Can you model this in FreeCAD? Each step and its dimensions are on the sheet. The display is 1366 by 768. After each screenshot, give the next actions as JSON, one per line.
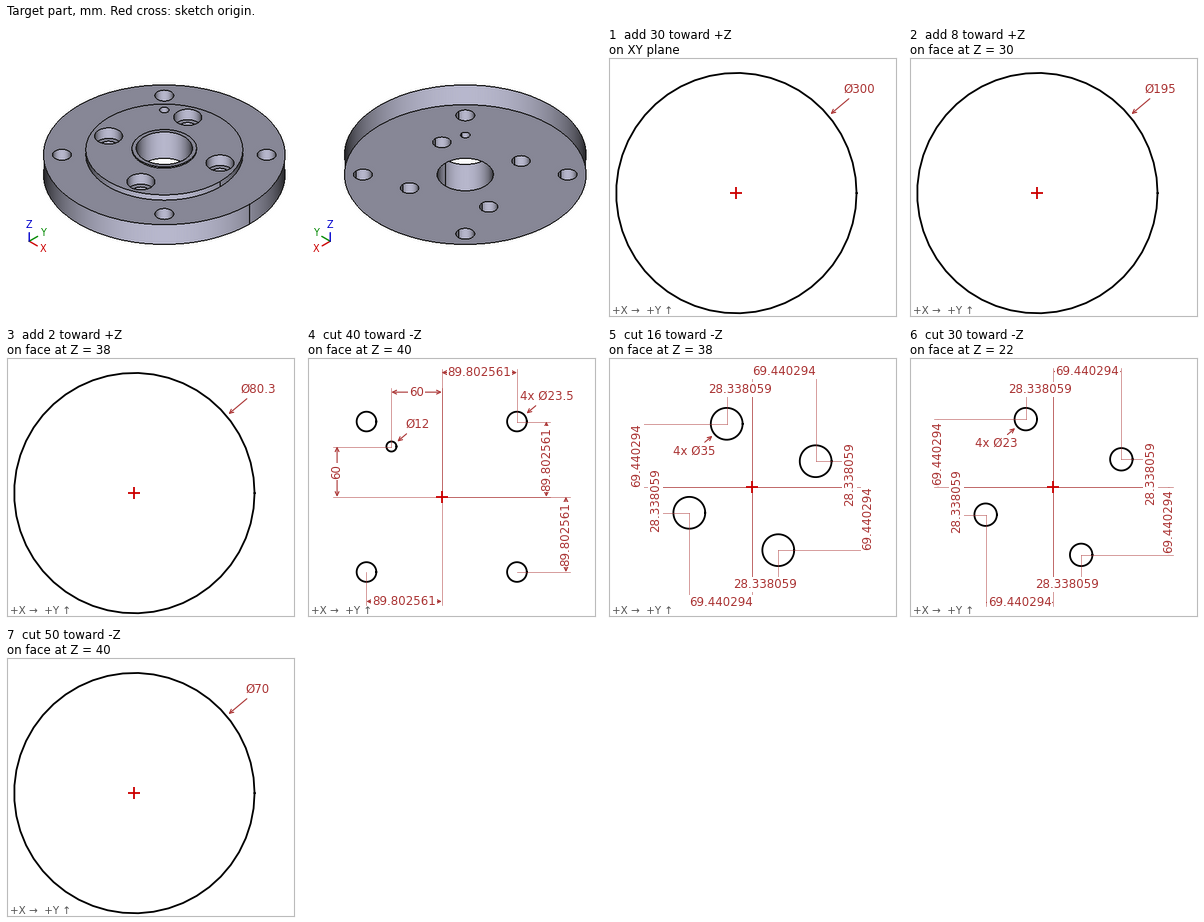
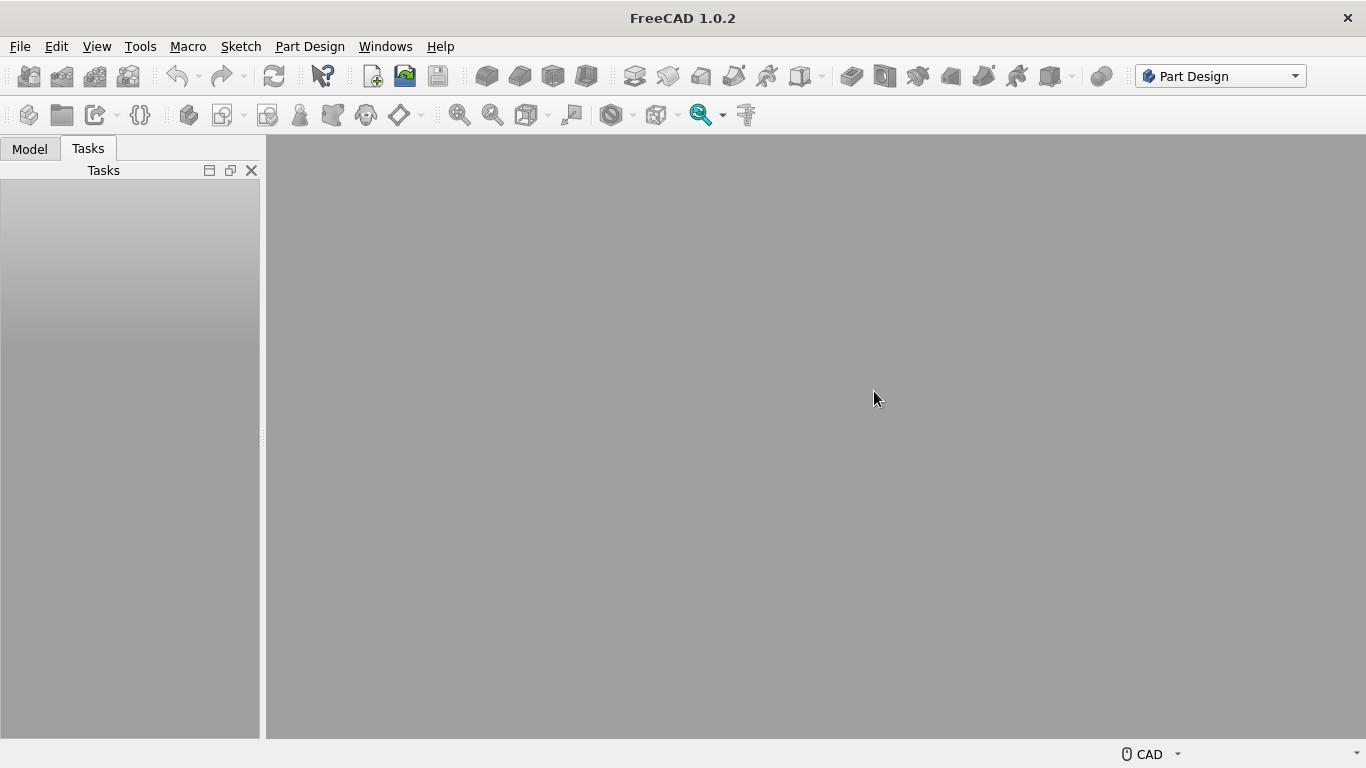
{"action": "left_click", "coordinate": [372, 76]}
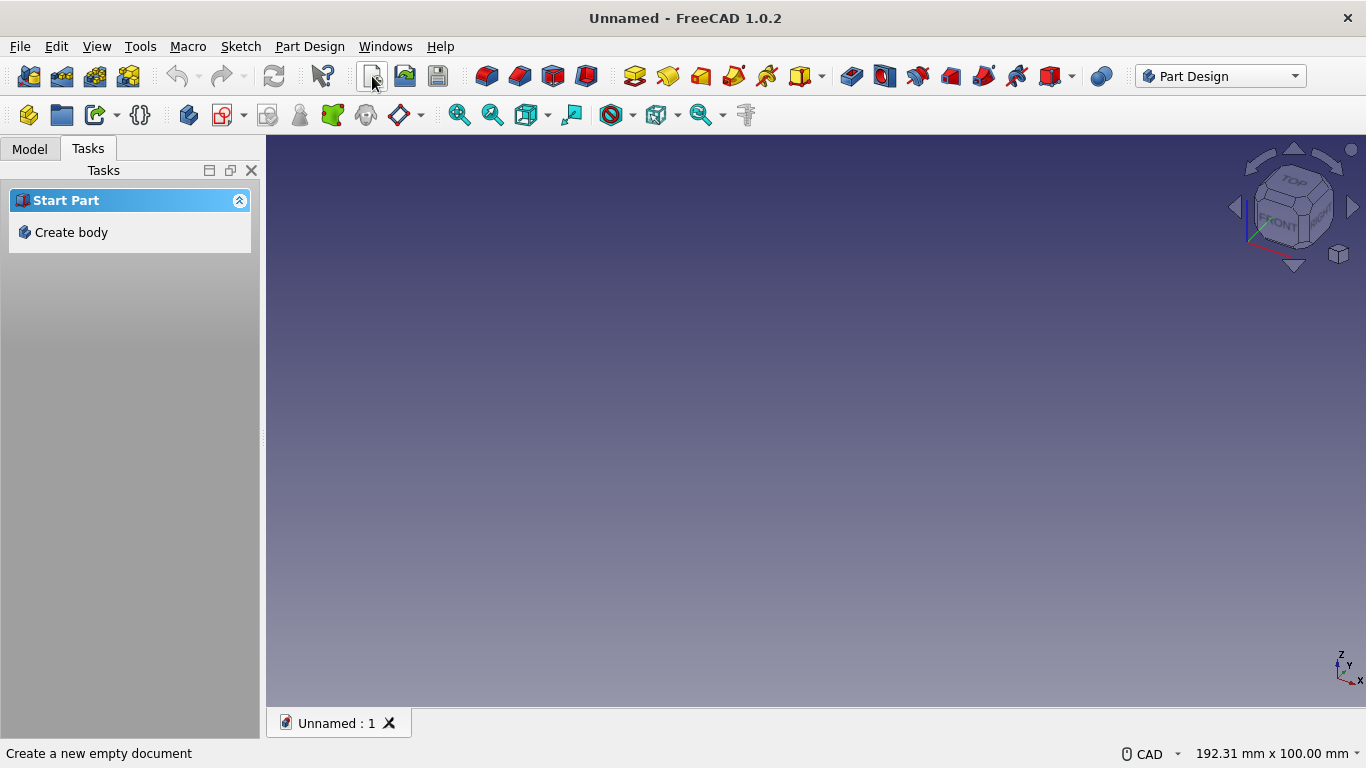
{"action": "left_click", "coordinate": [222, 116]}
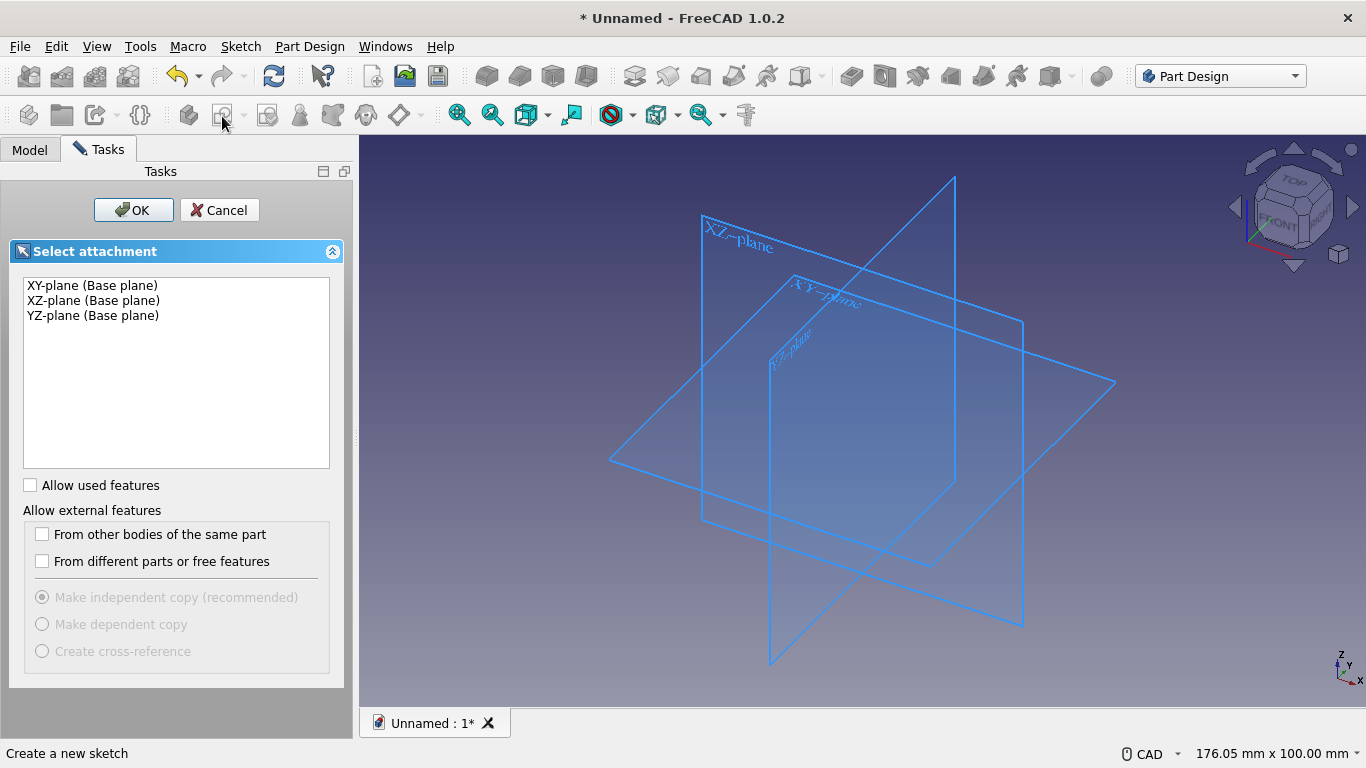
{"action": "left_click", "coordinate": [84, 286]}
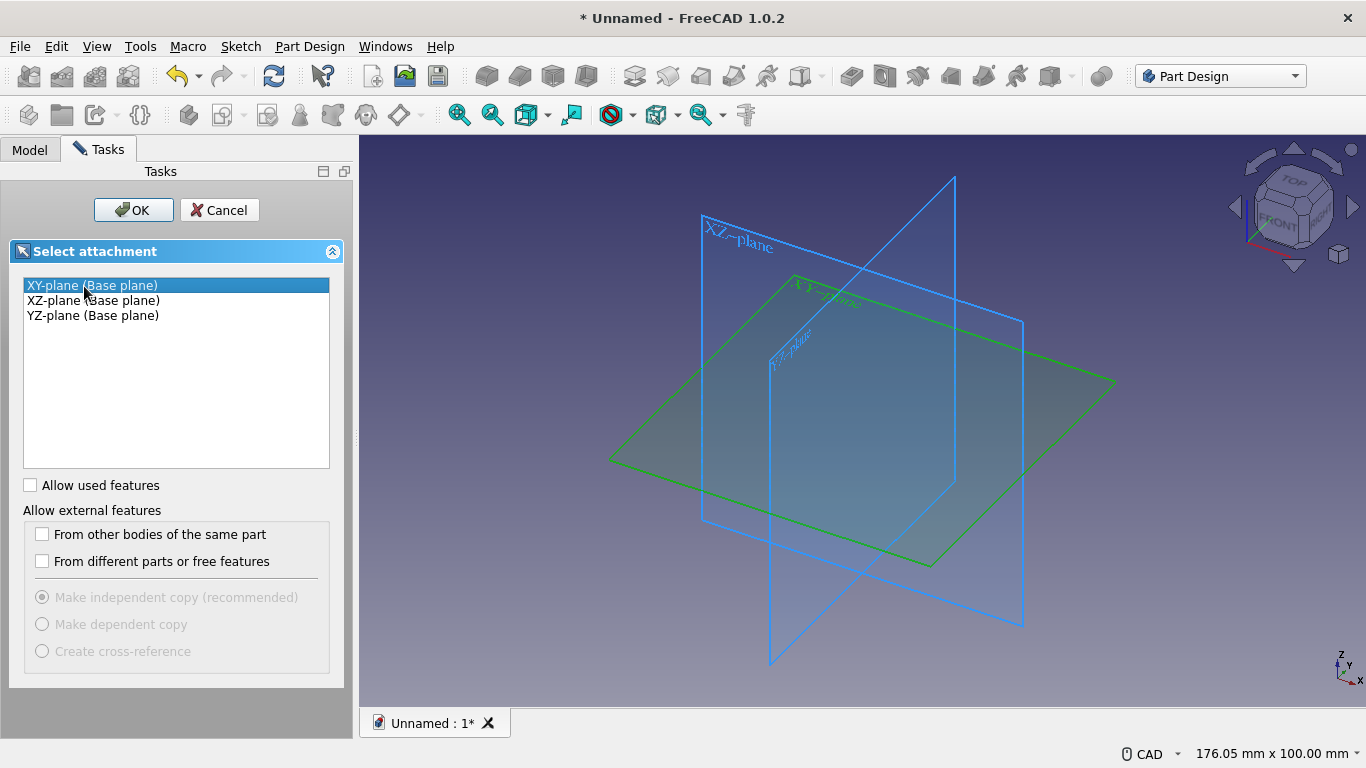
{"action": "left_click", "coordinate": [134, 210]}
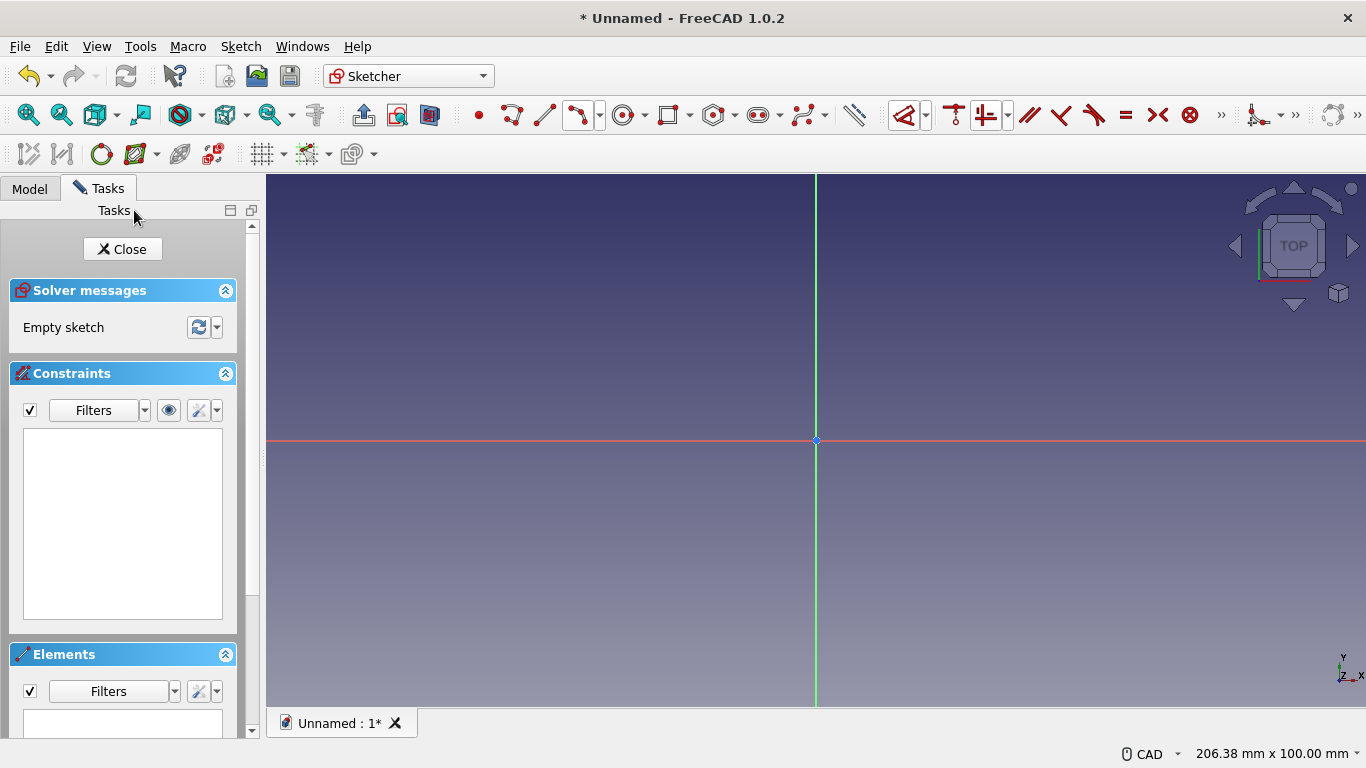
{"action": "scroll", "coordinate": [730, 440], "scroll_direction": "down", "scroll_amount": 8}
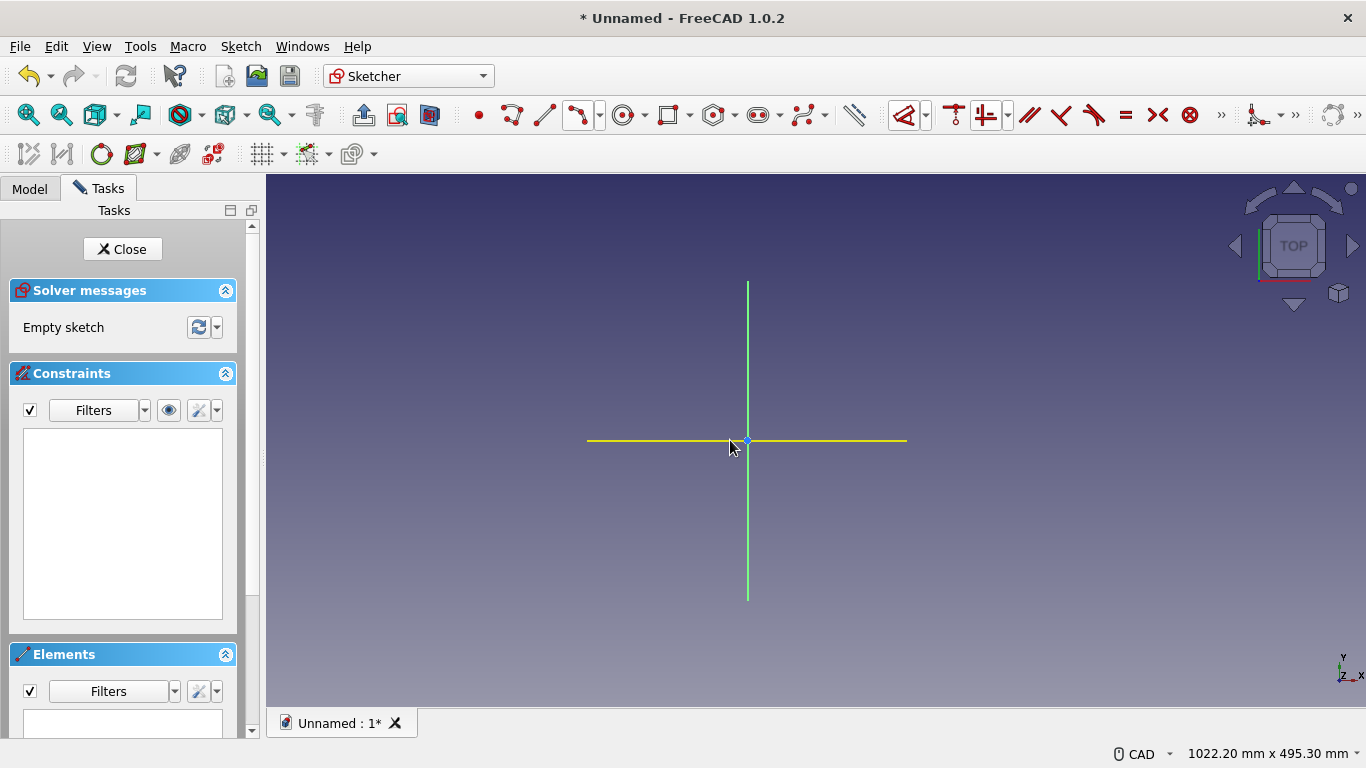
{"action": "key", "text": "g c"}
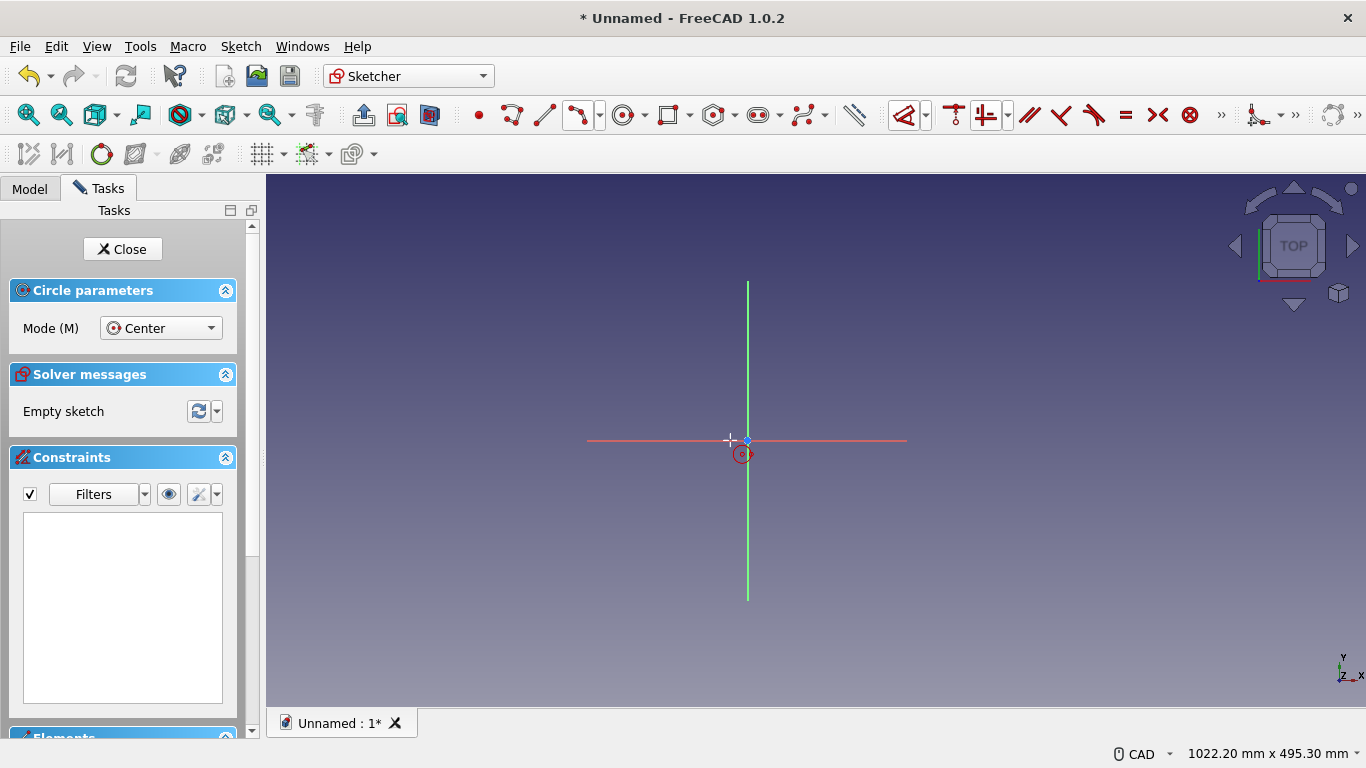
{"action": "left_click", "coordinate": [748, 440]}
{"action": "left_click", "coordinate": [862, 326]}
{"action": "key", "text": "Escape"}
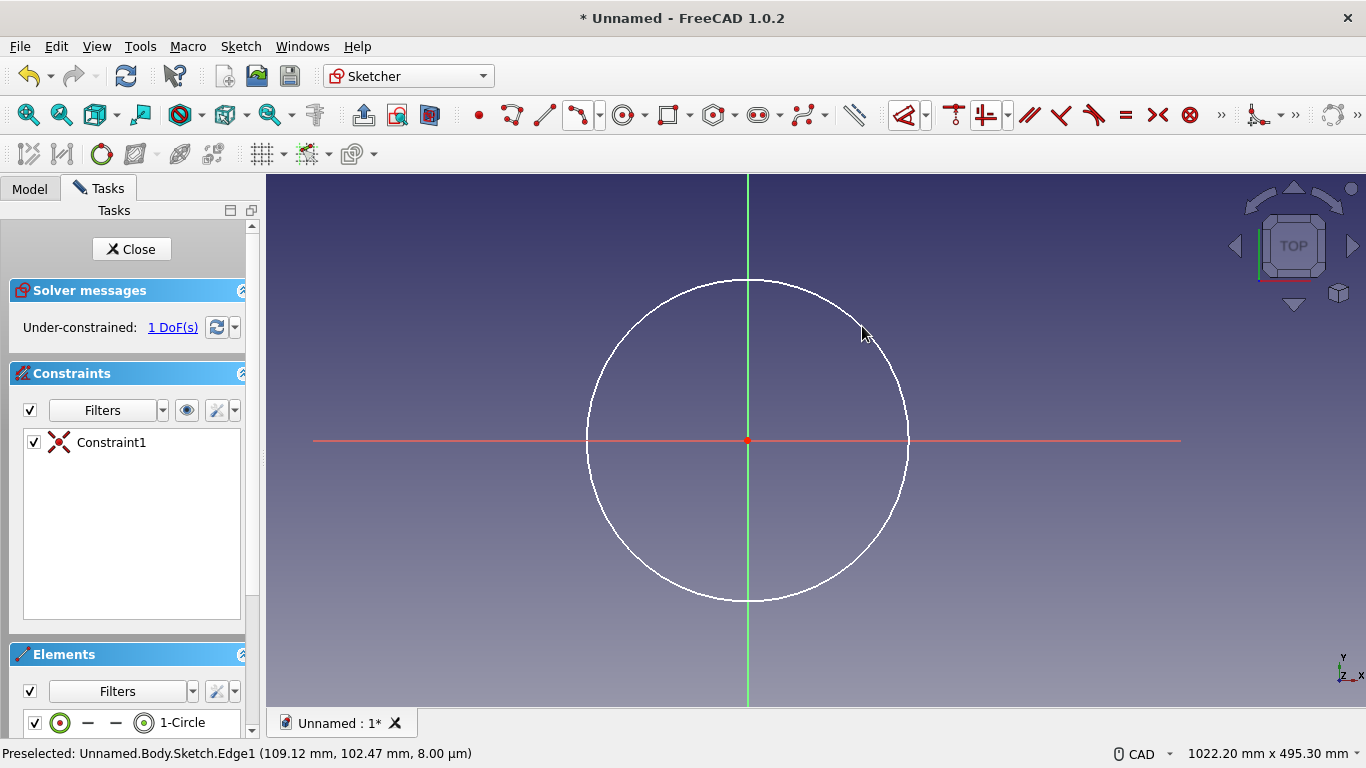
{"action": "key", "text": "d"}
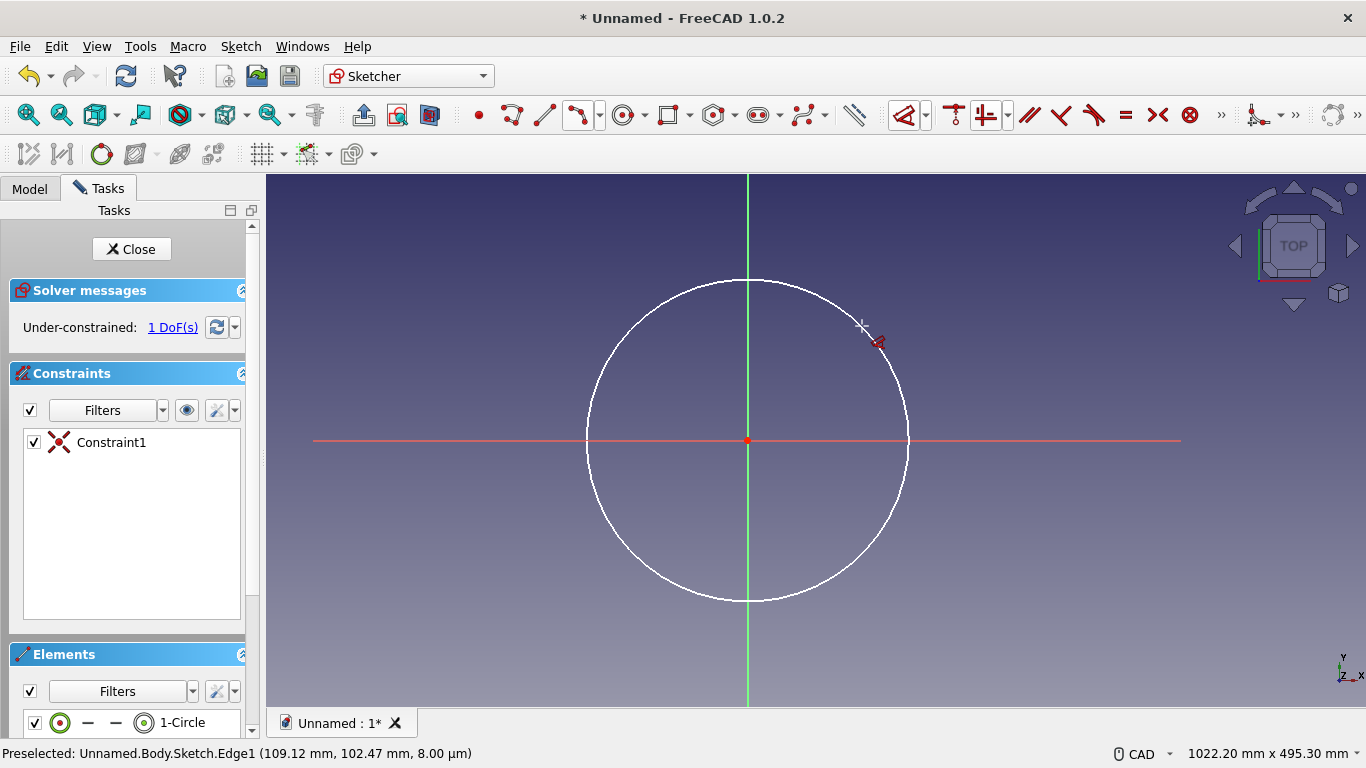
{"action": "left_click", "coordinate": [861, 326]}
{"action": "left_click", "coordinate": [884, 303]}